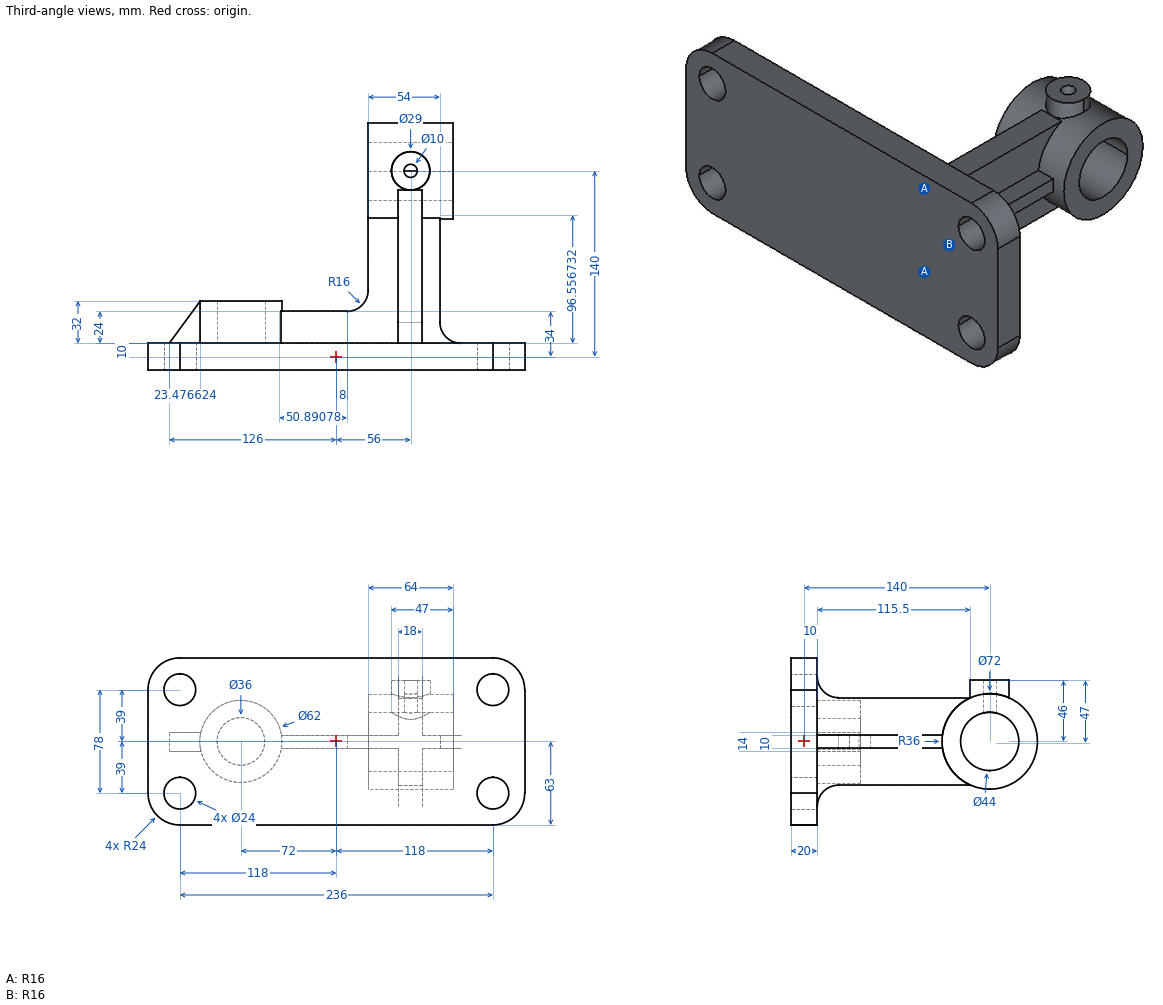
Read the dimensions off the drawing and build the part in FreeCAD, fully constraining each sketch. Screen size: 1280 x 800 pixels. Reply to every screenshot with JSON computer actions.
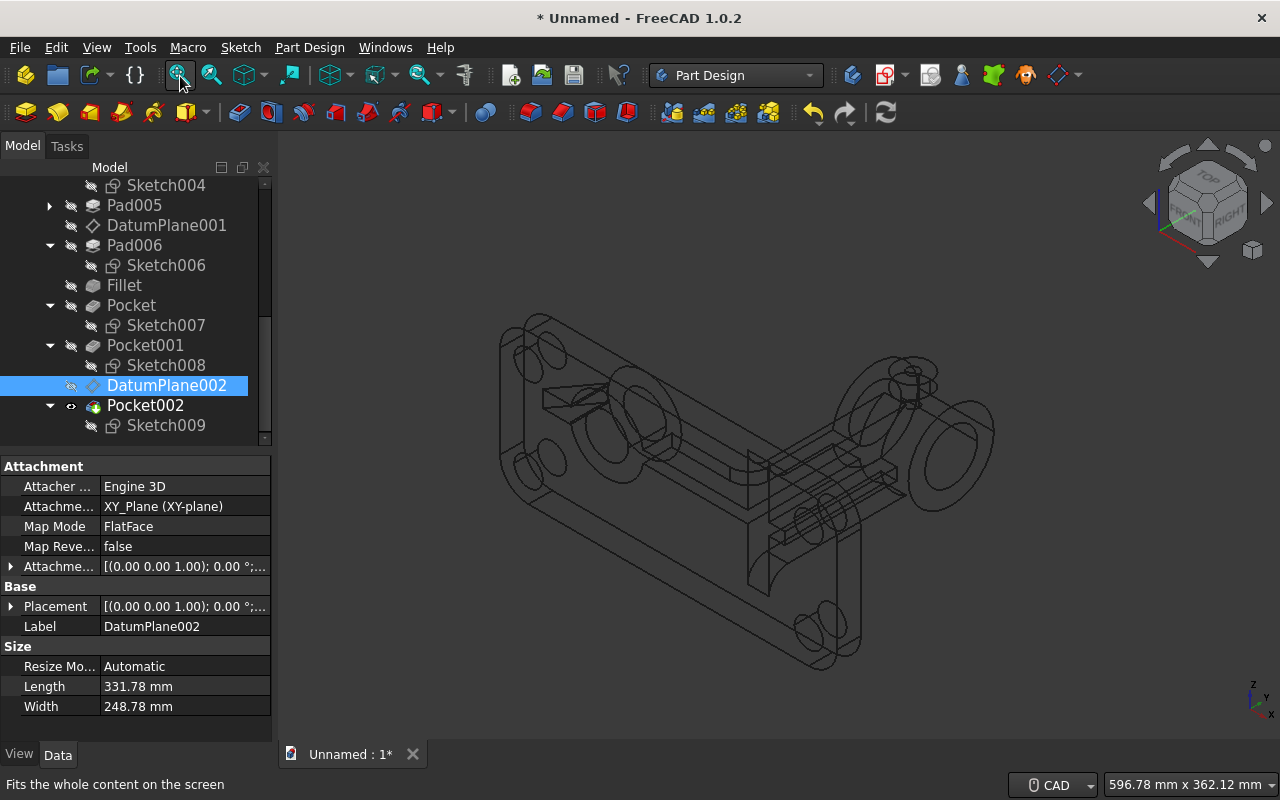
{"action": "left_click", "coordinate": [785, 538]}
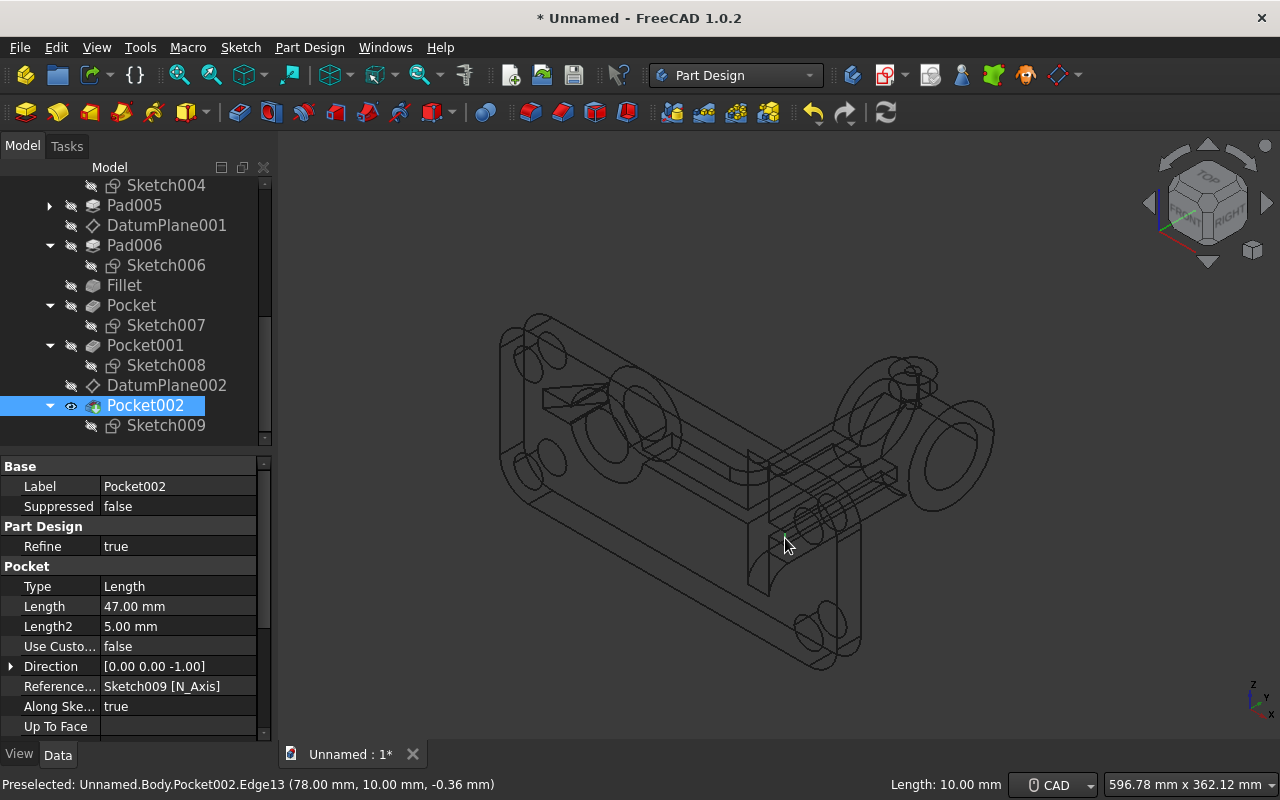
{"action": "key", "text": "v 1"}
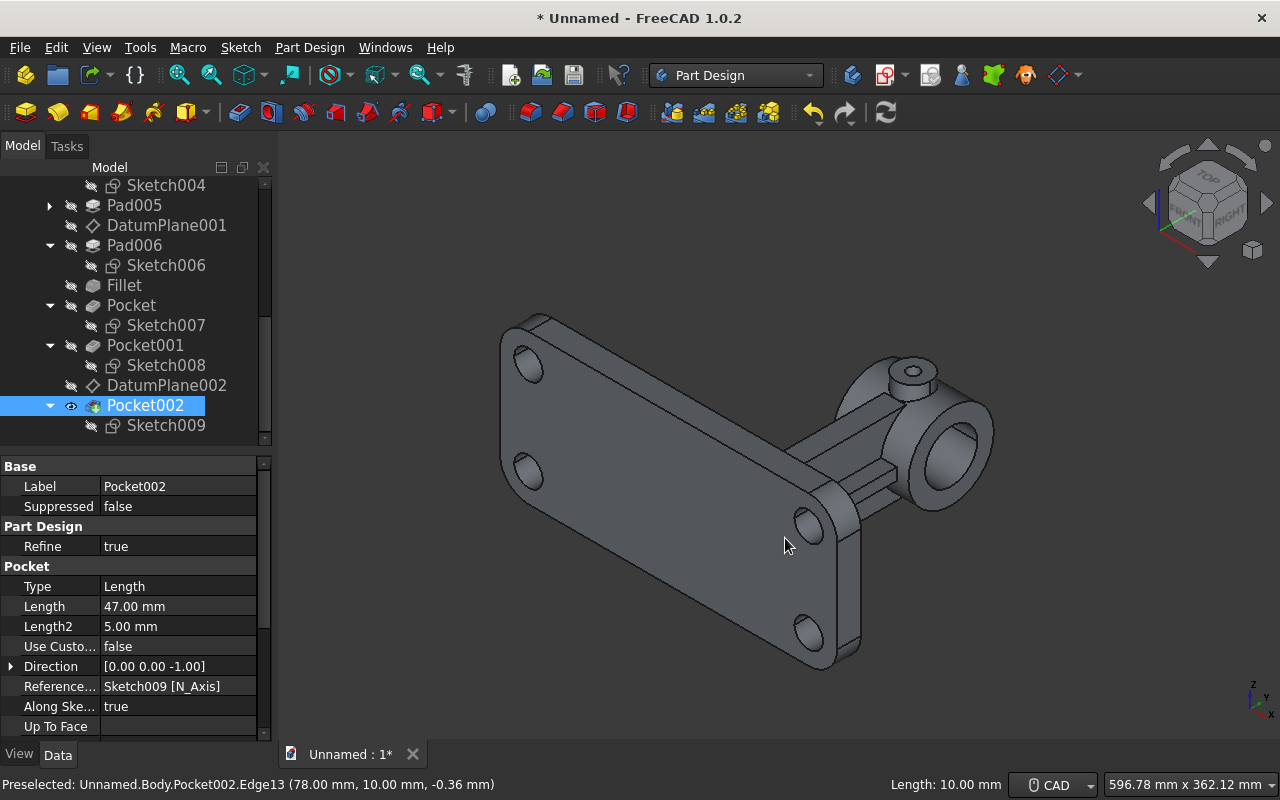
{"action": "left_click", "coordinate": [532, 112]}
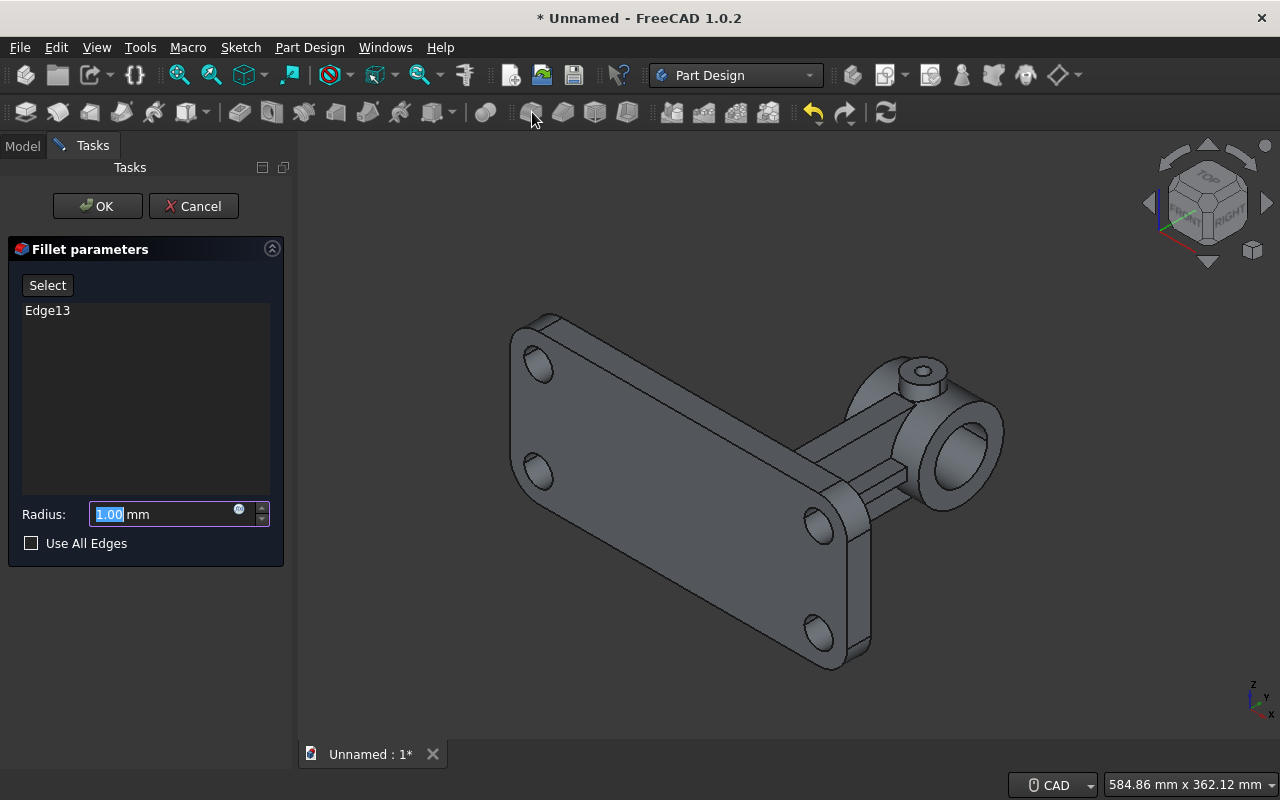
{"action": "type", "text": "16"}
{"action": "key", "text": "Tab"}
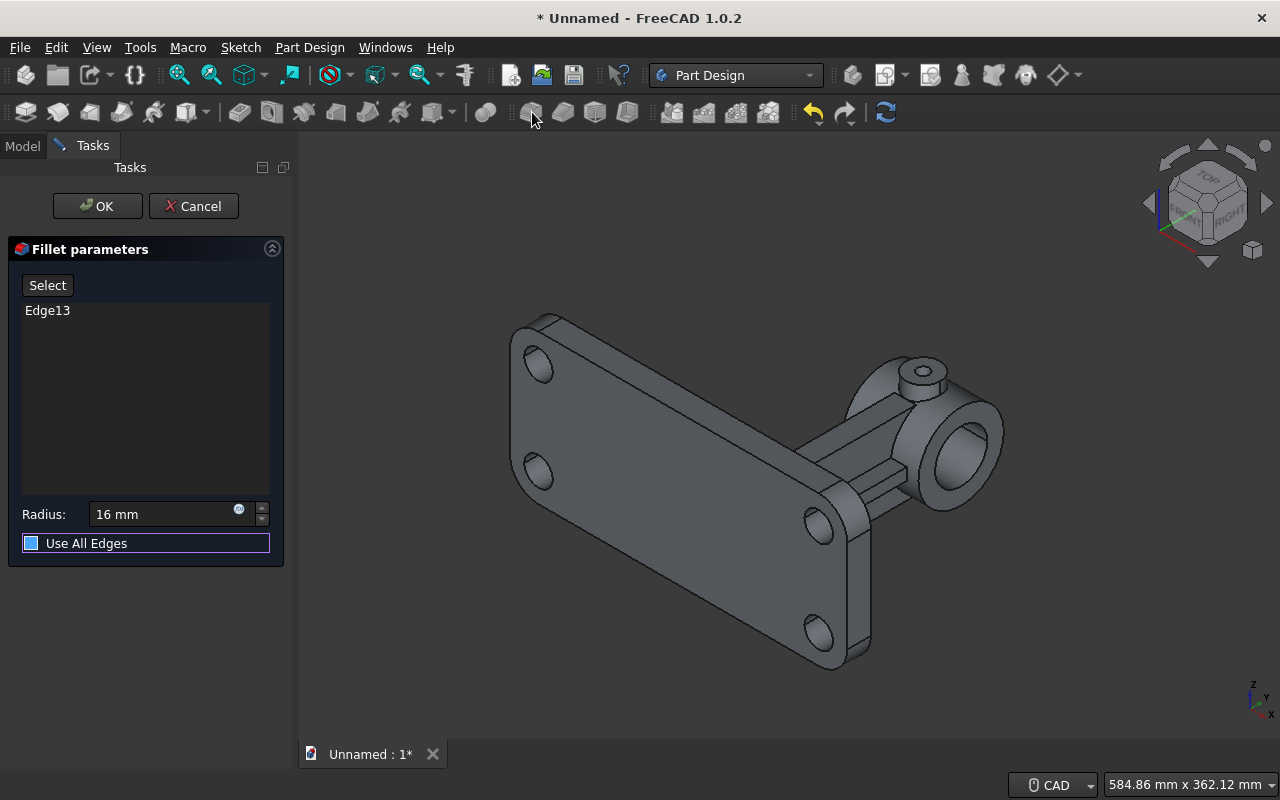
{"action": "left_click", "coordinate": [98, 206]}